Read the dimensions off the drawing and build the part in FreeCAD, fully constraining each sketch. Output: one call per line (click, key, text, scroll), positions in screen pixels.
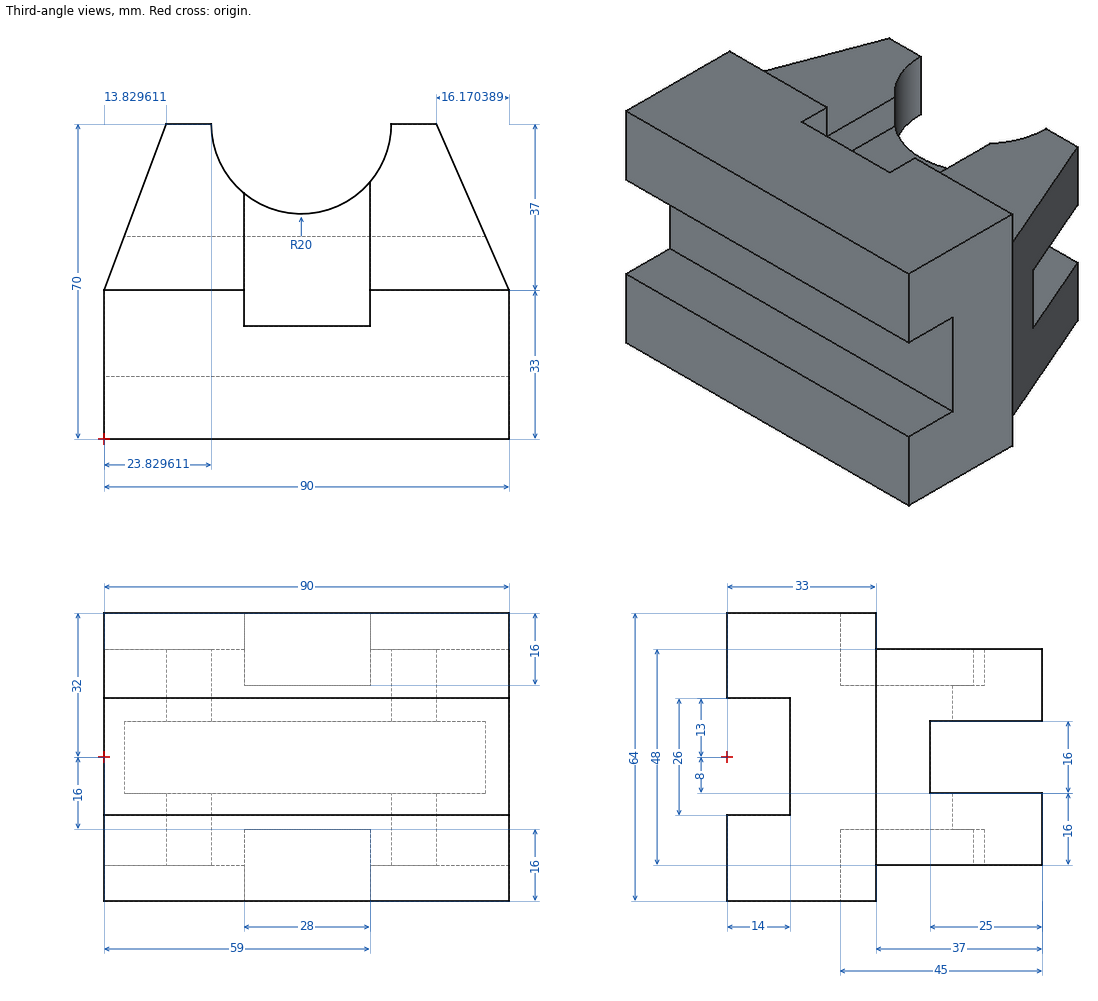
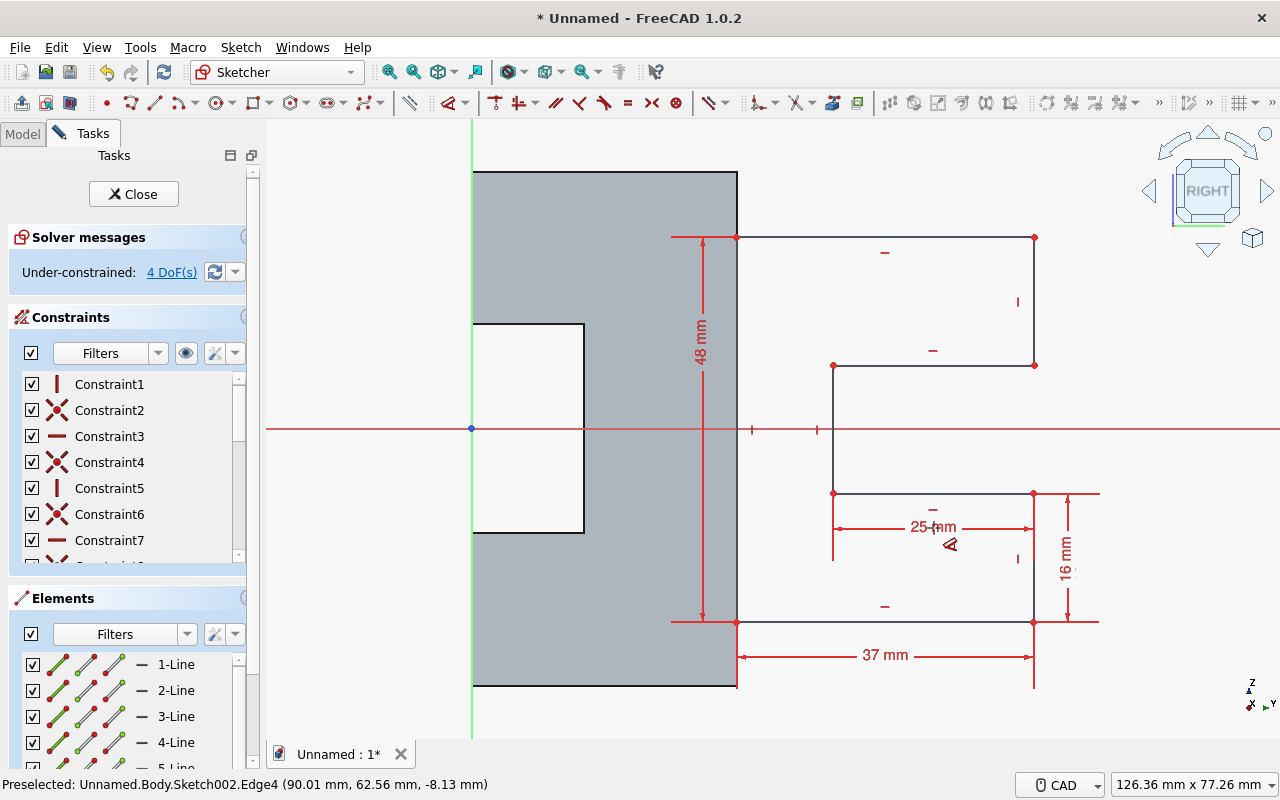
click(833, 456)
click(867, 401)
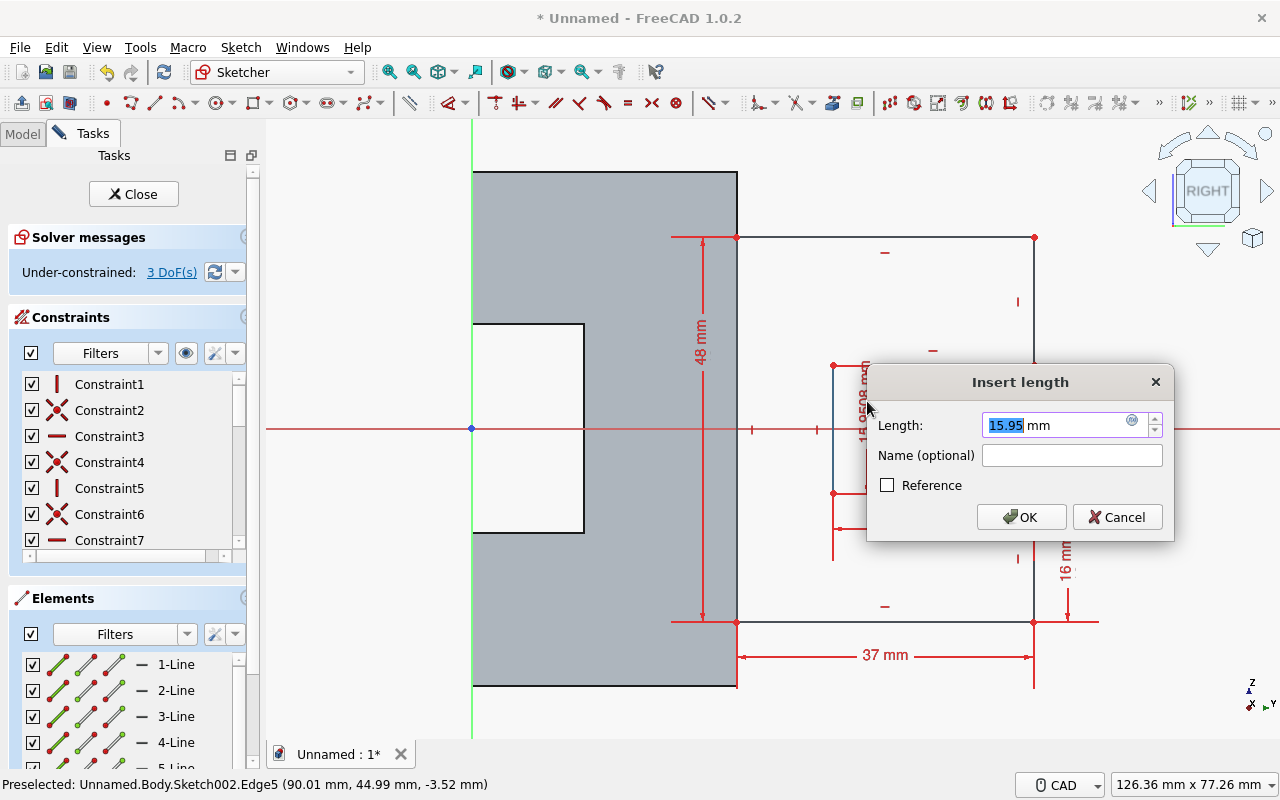
text(16)
key(Return)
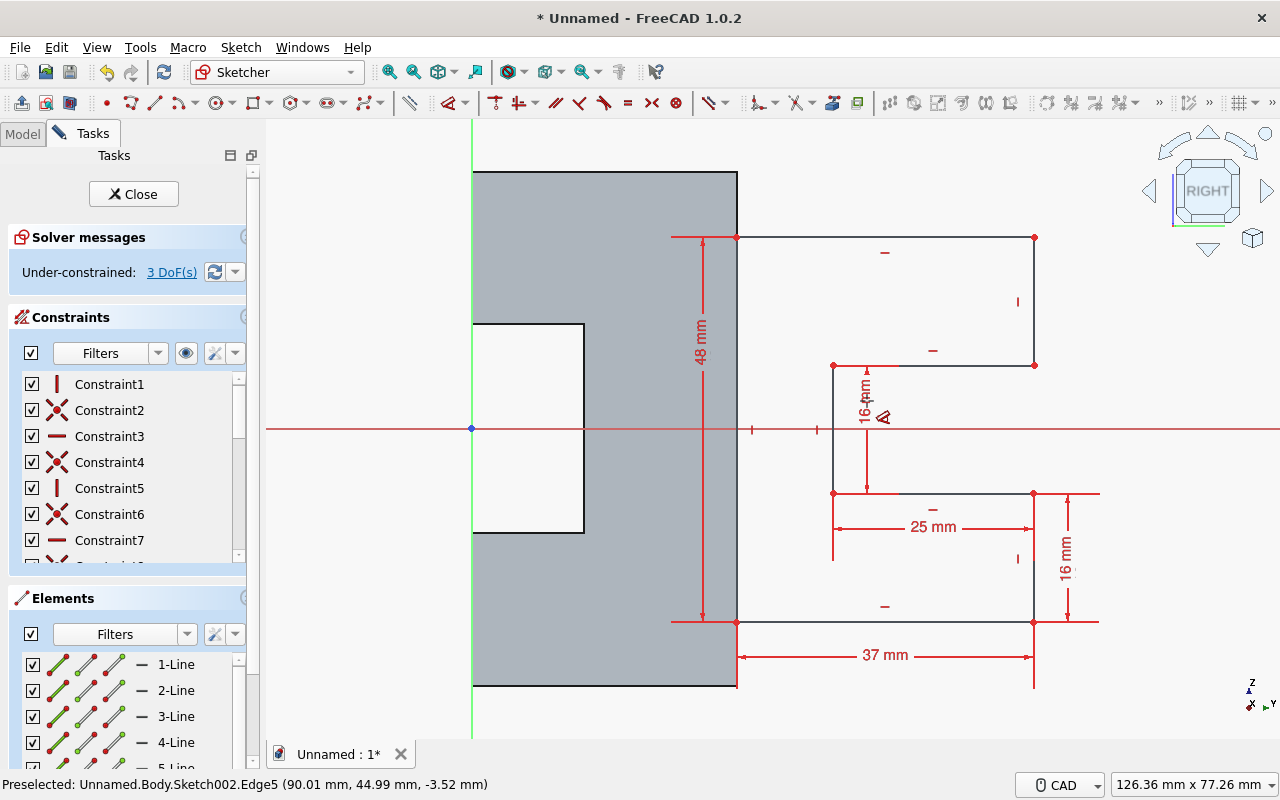
click(893, 366)
click(934, 332)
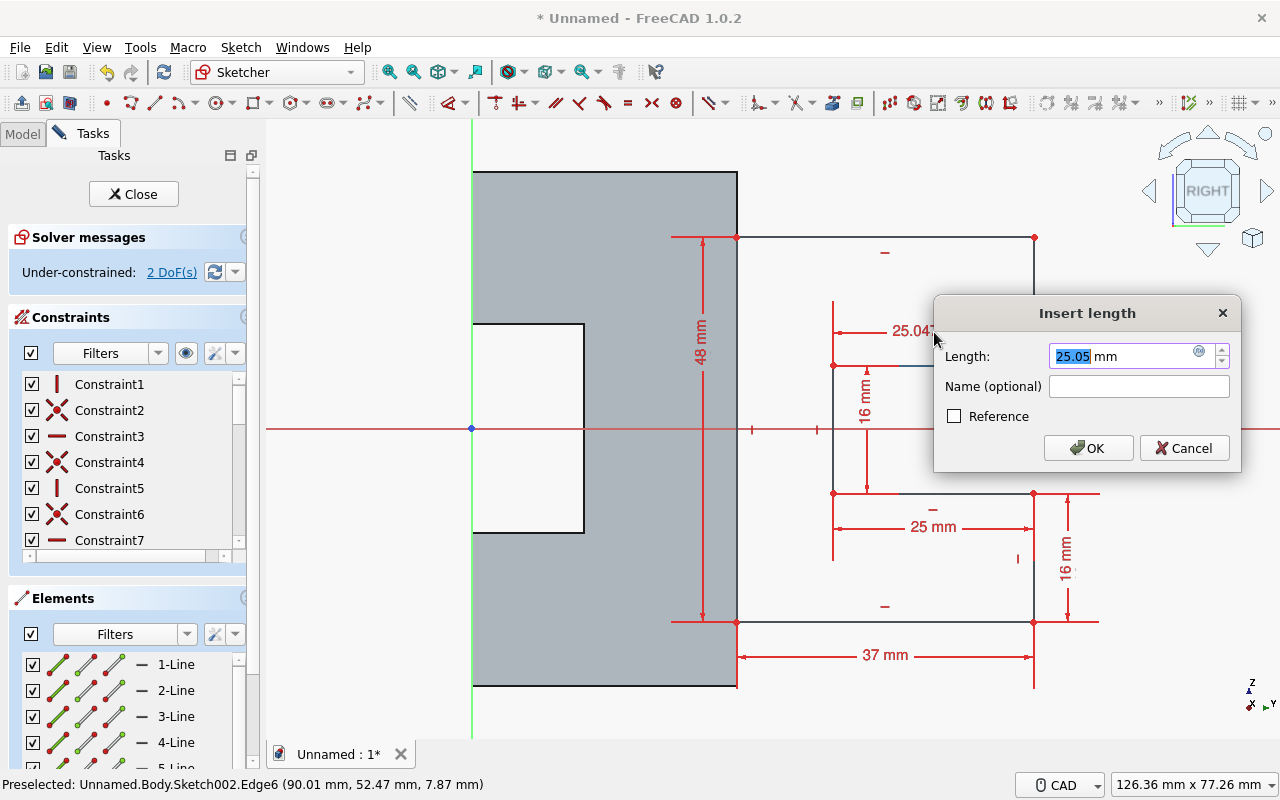
text(25)
key(Return)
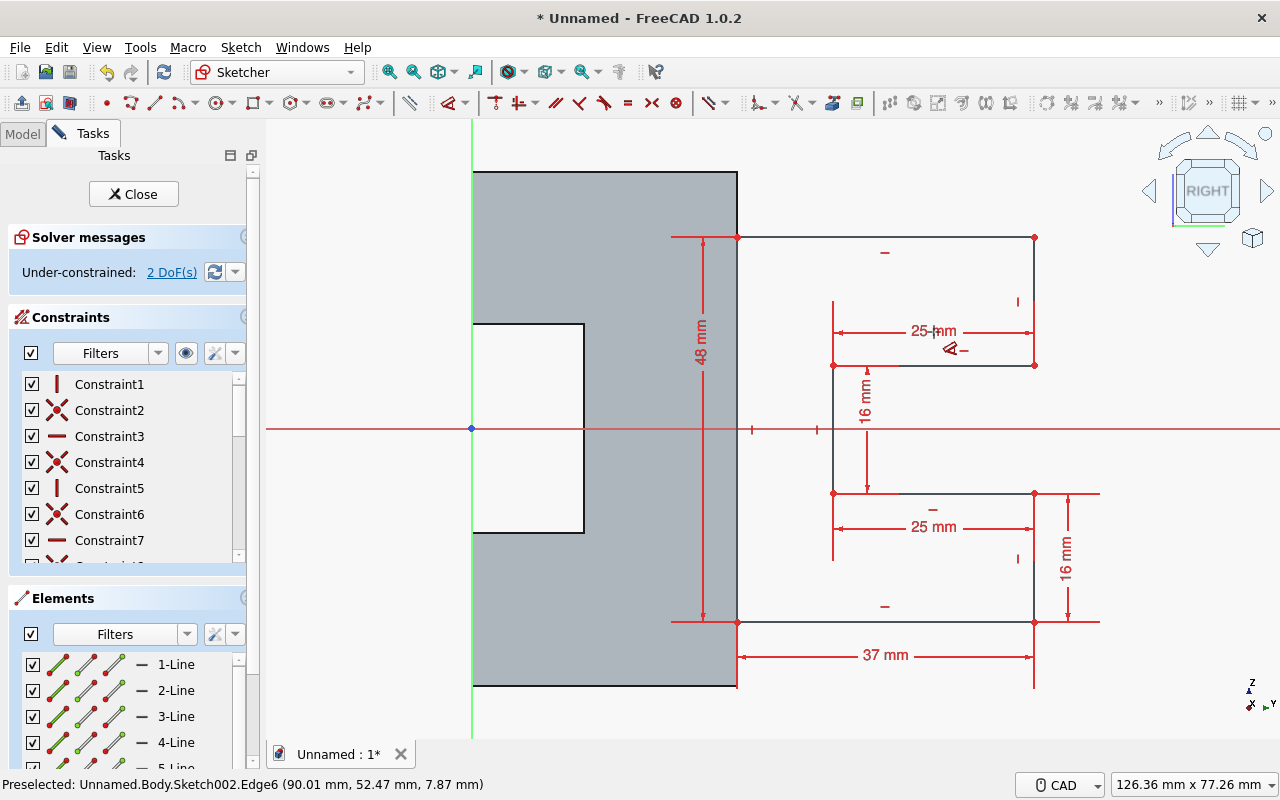
click(1034, 494)
click(1068, 461)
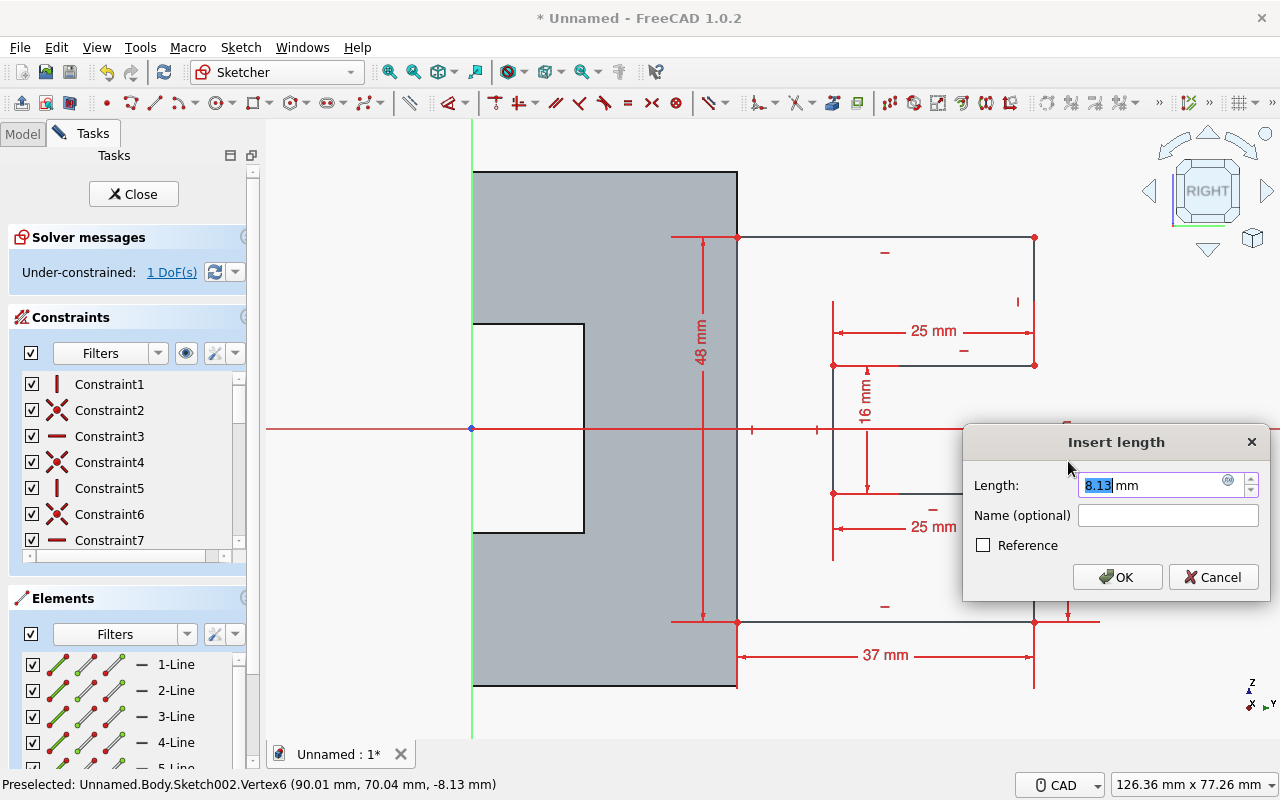
text(8)
key(Return)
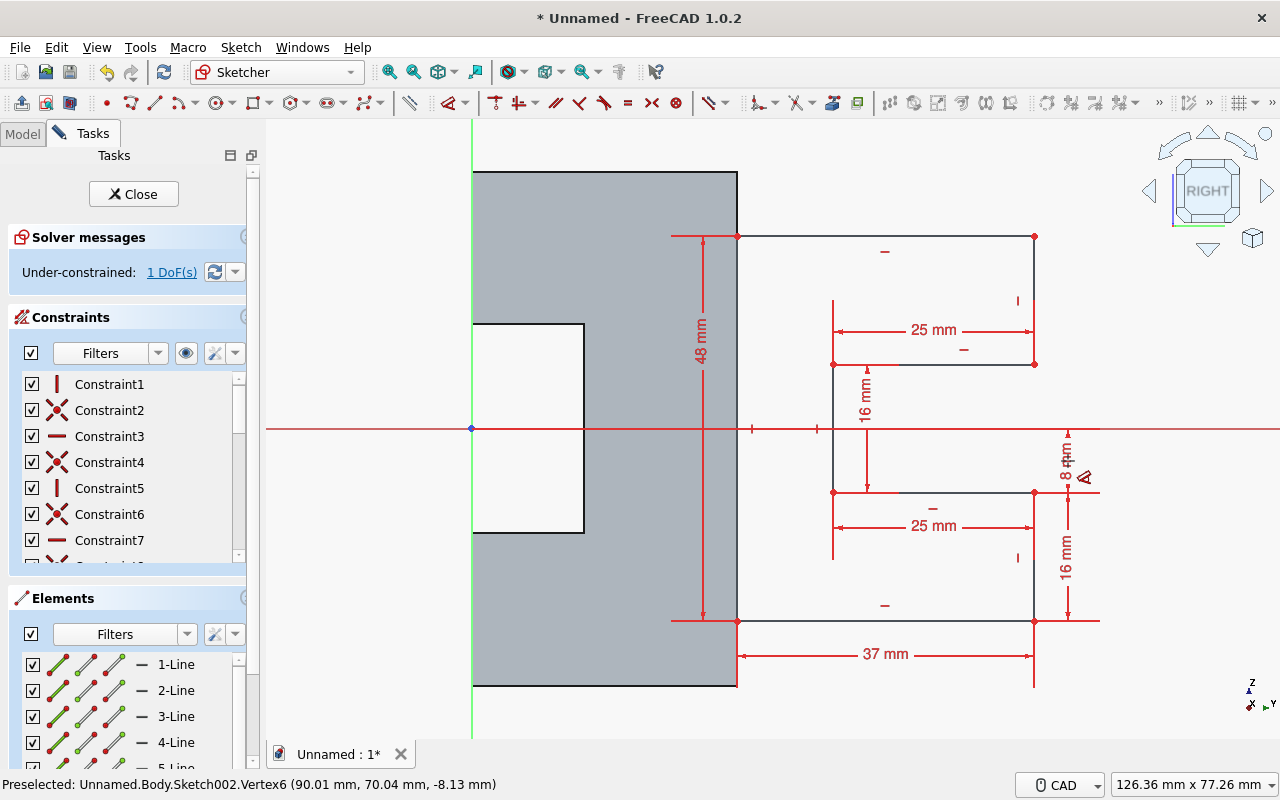
click(737, 236)
click(605, 202)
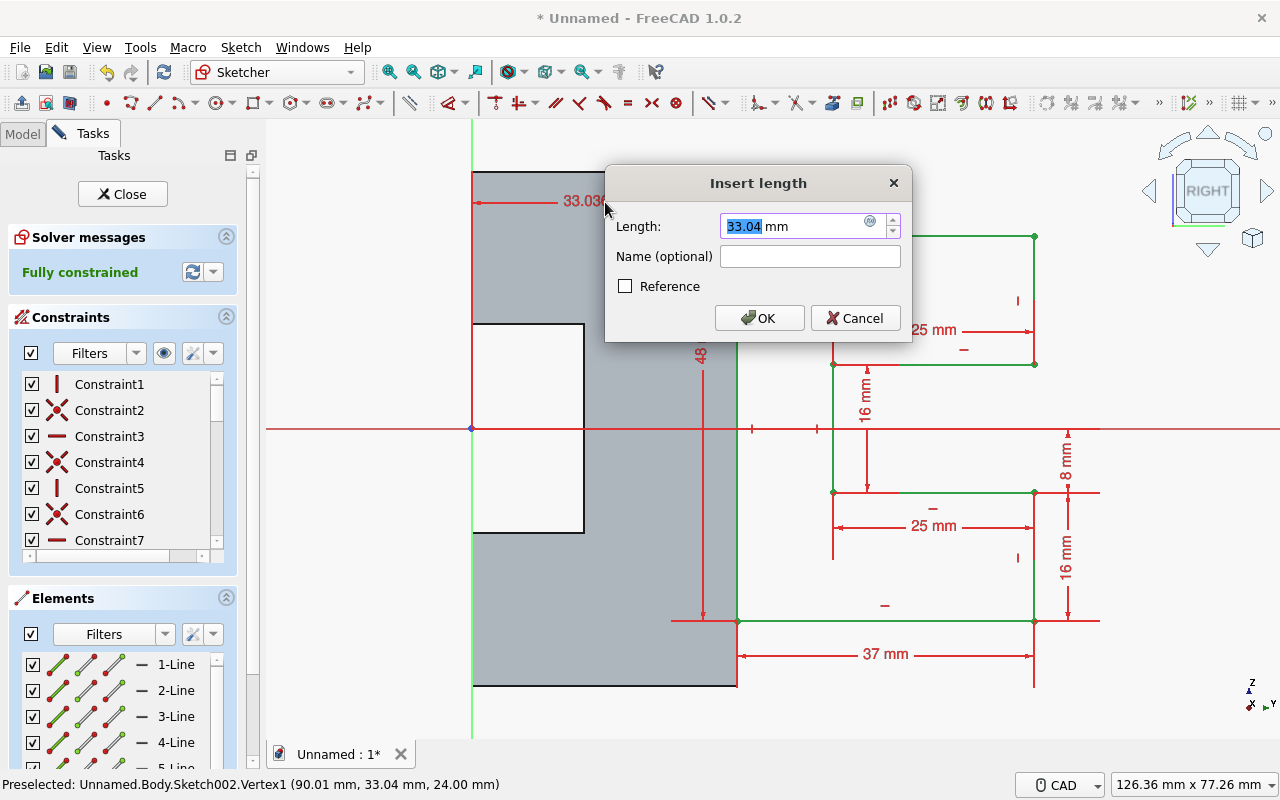
text(33)
key(Return)
key(Escape)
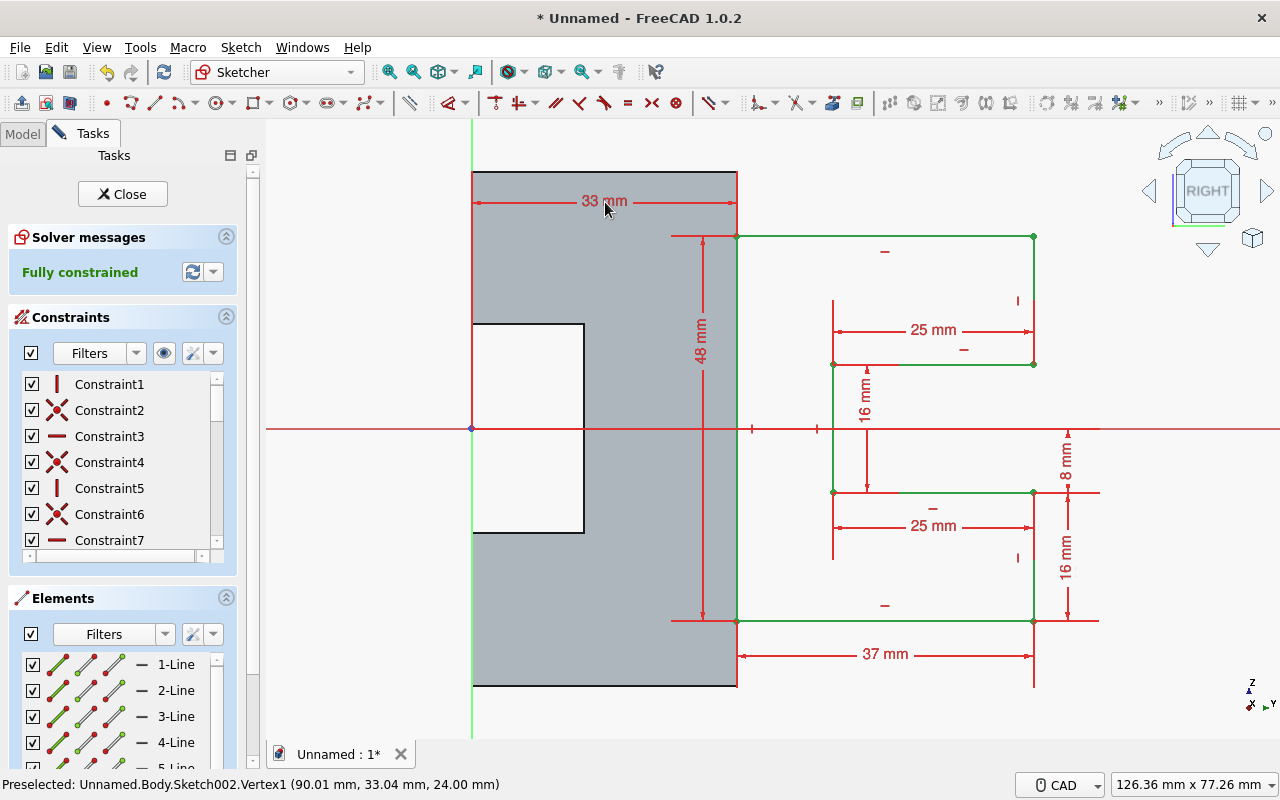
click(123, 194)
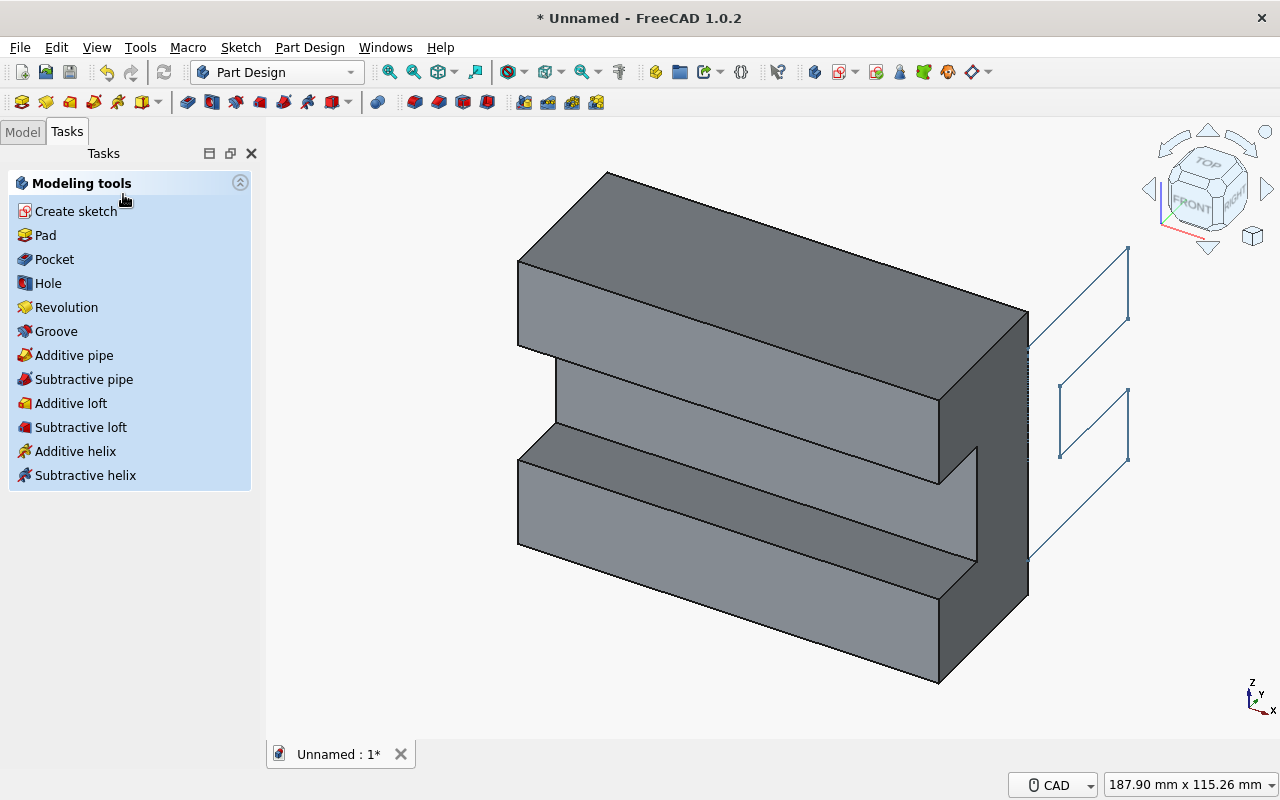
click(22, 102)